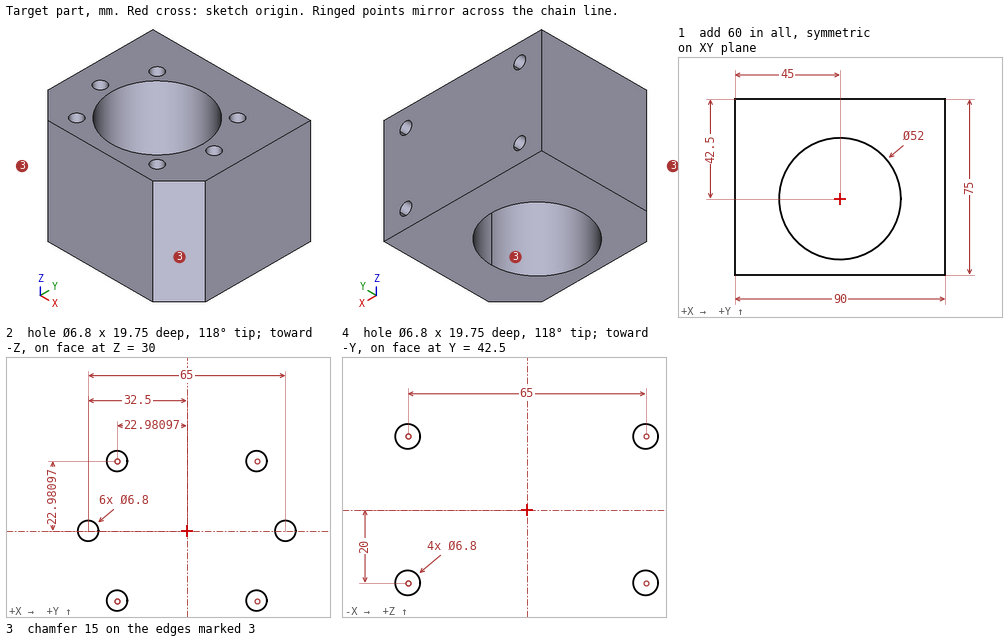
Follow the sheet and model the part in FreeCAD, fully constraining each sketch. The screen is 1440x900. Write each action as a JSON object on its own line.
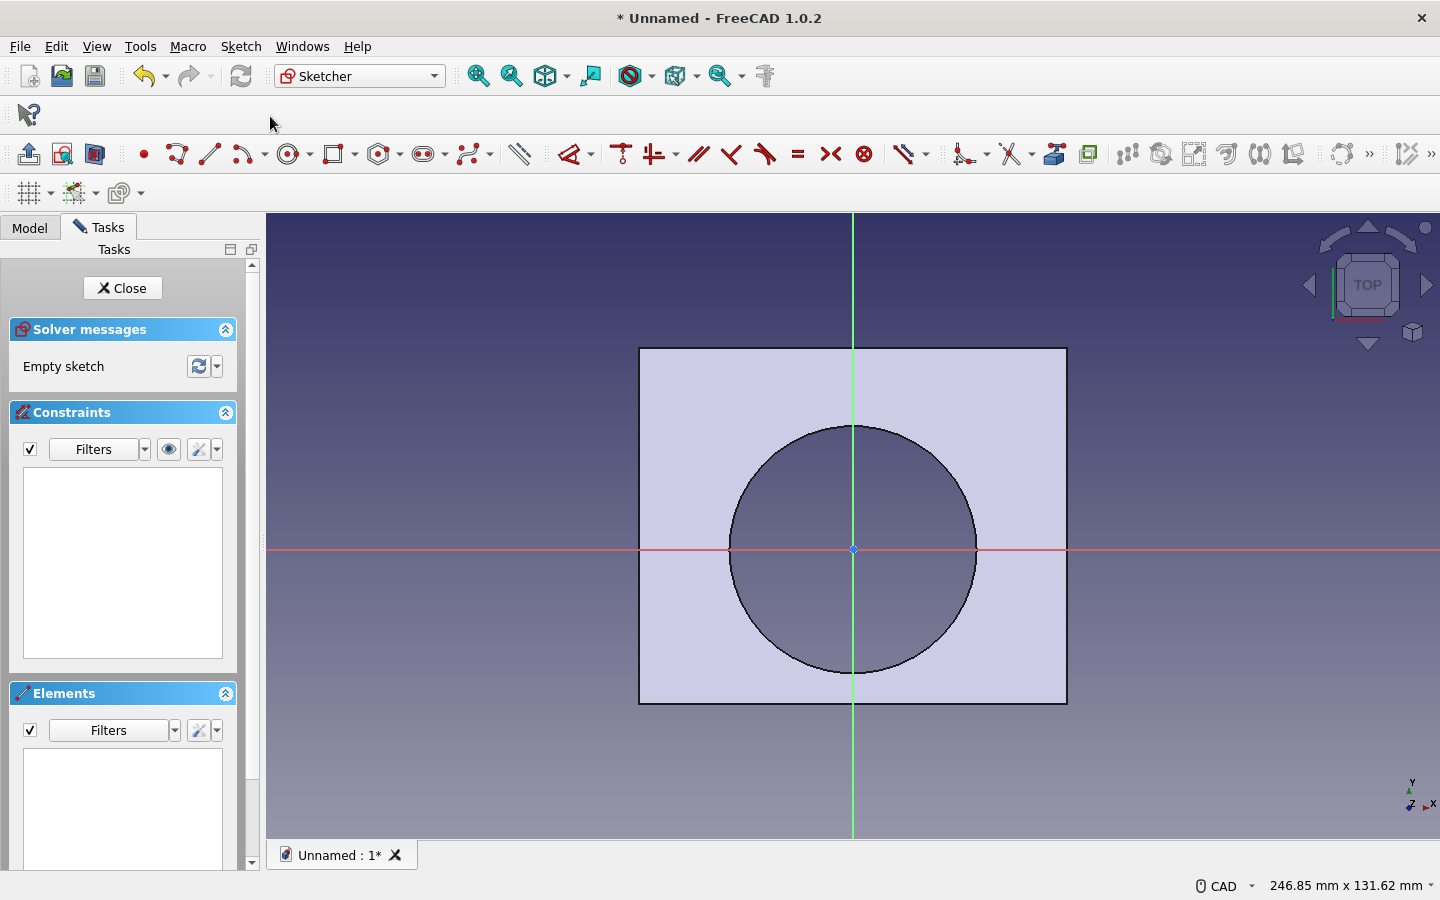
{"action": "scroll", "coordinate": [992, 598], "scroll_direction": "up", "scroll_amount": 2}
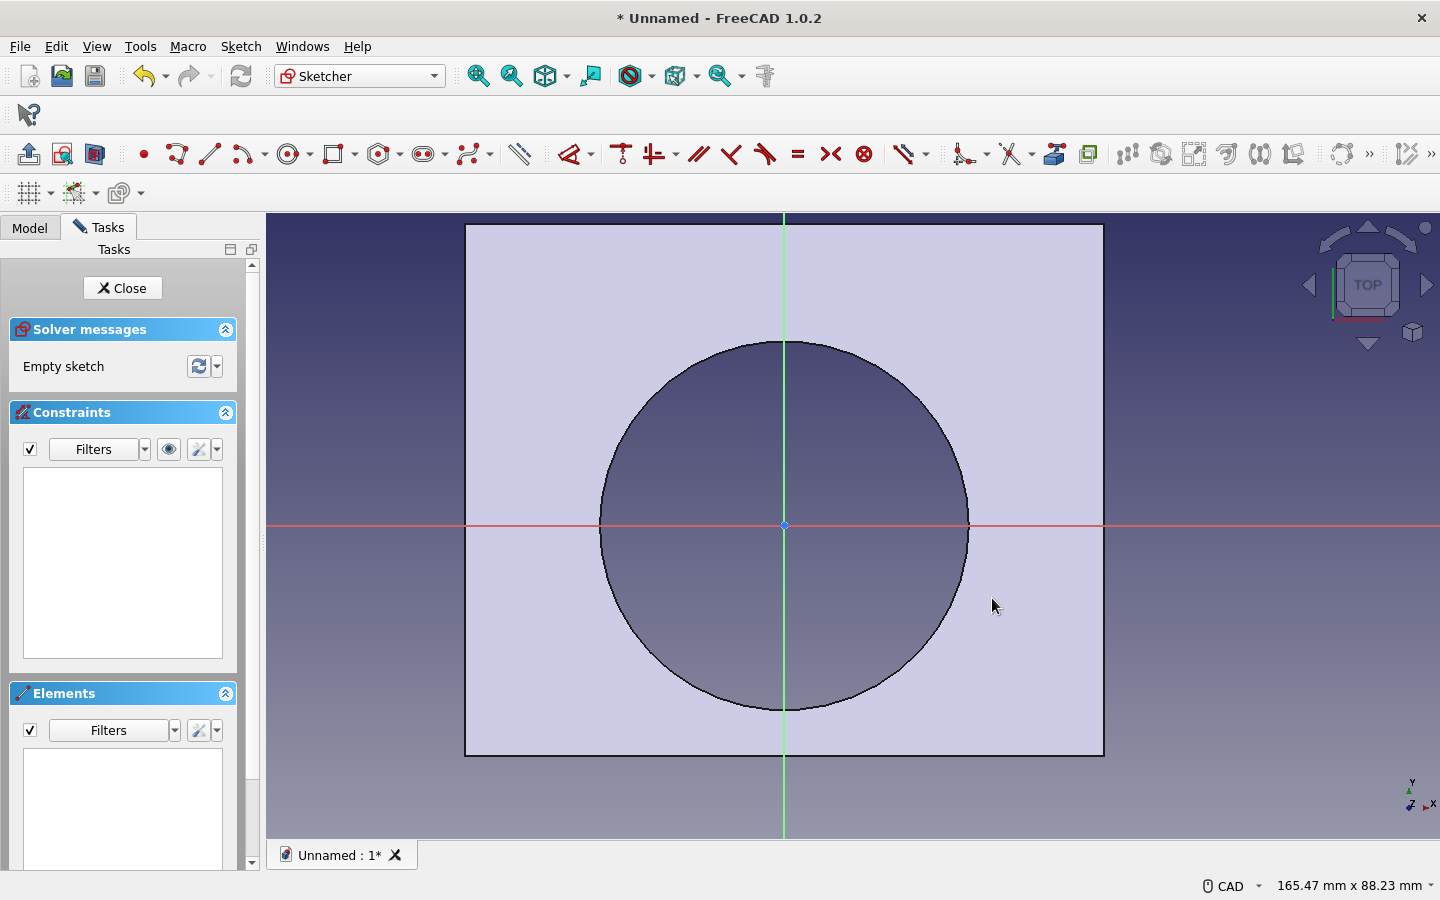
{"action": "left_click", "coordinate": [288, 154]}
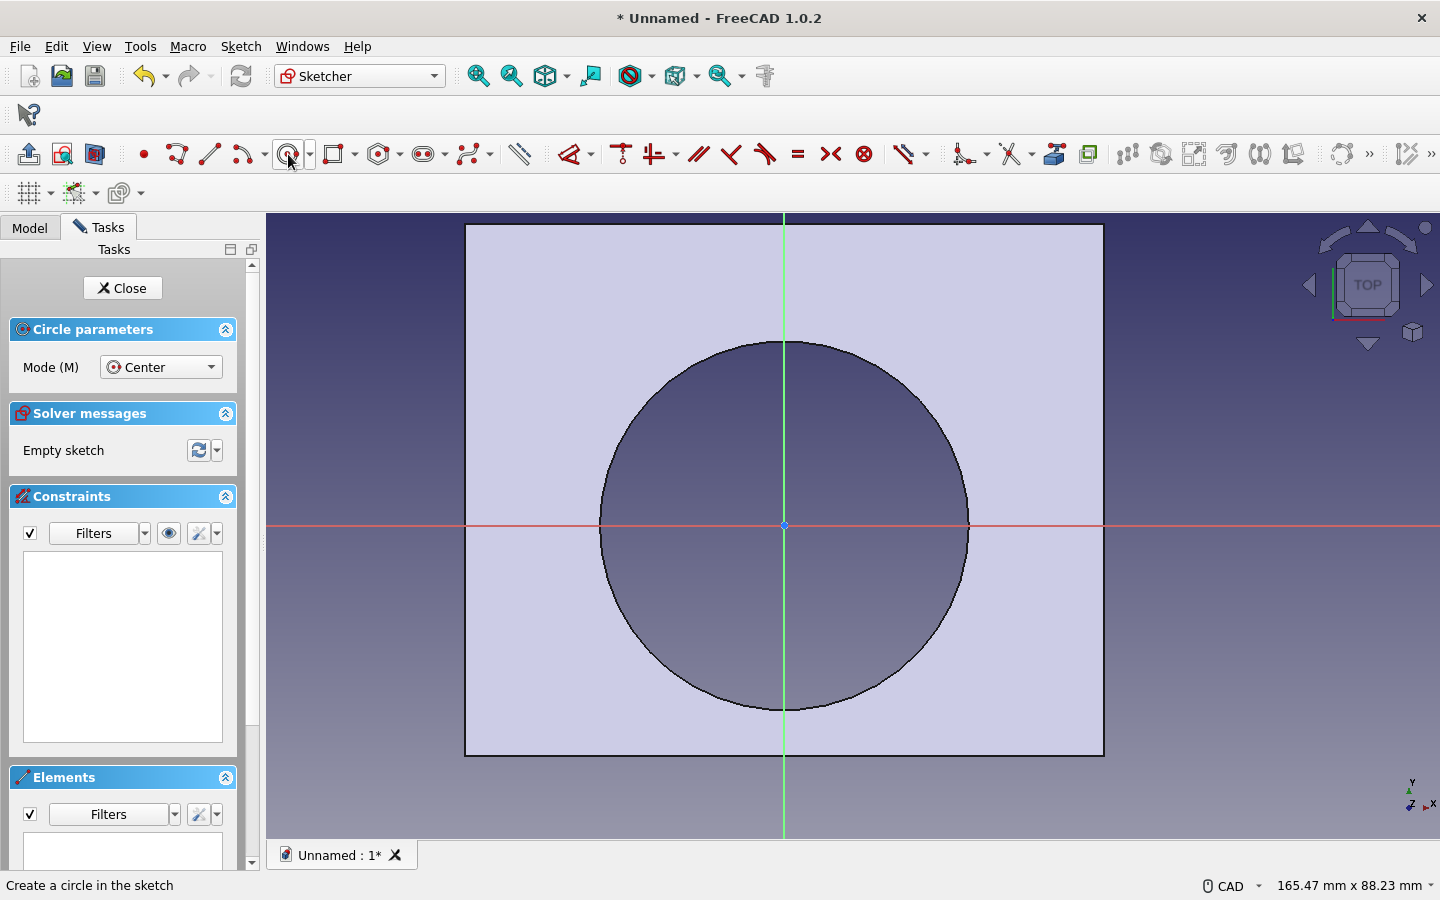
{"action": "left_click", "coordinate": [554, 526]}
{"action": "mouse_move", "coordinate": [571, 509]}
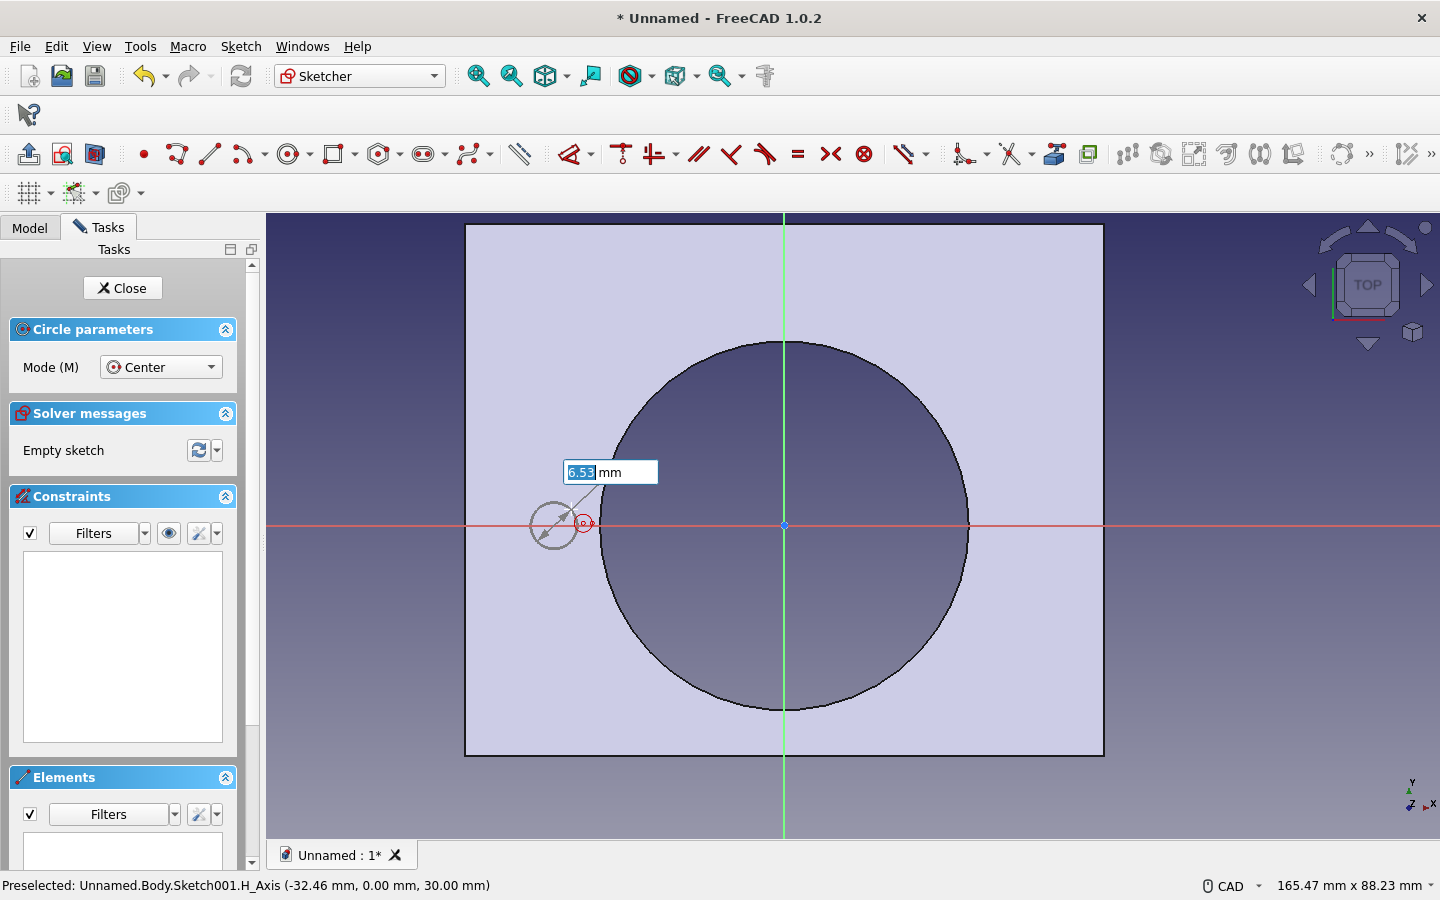
{"action": "type", "text": "6.8"}
{"action": "key", "text": "Return"}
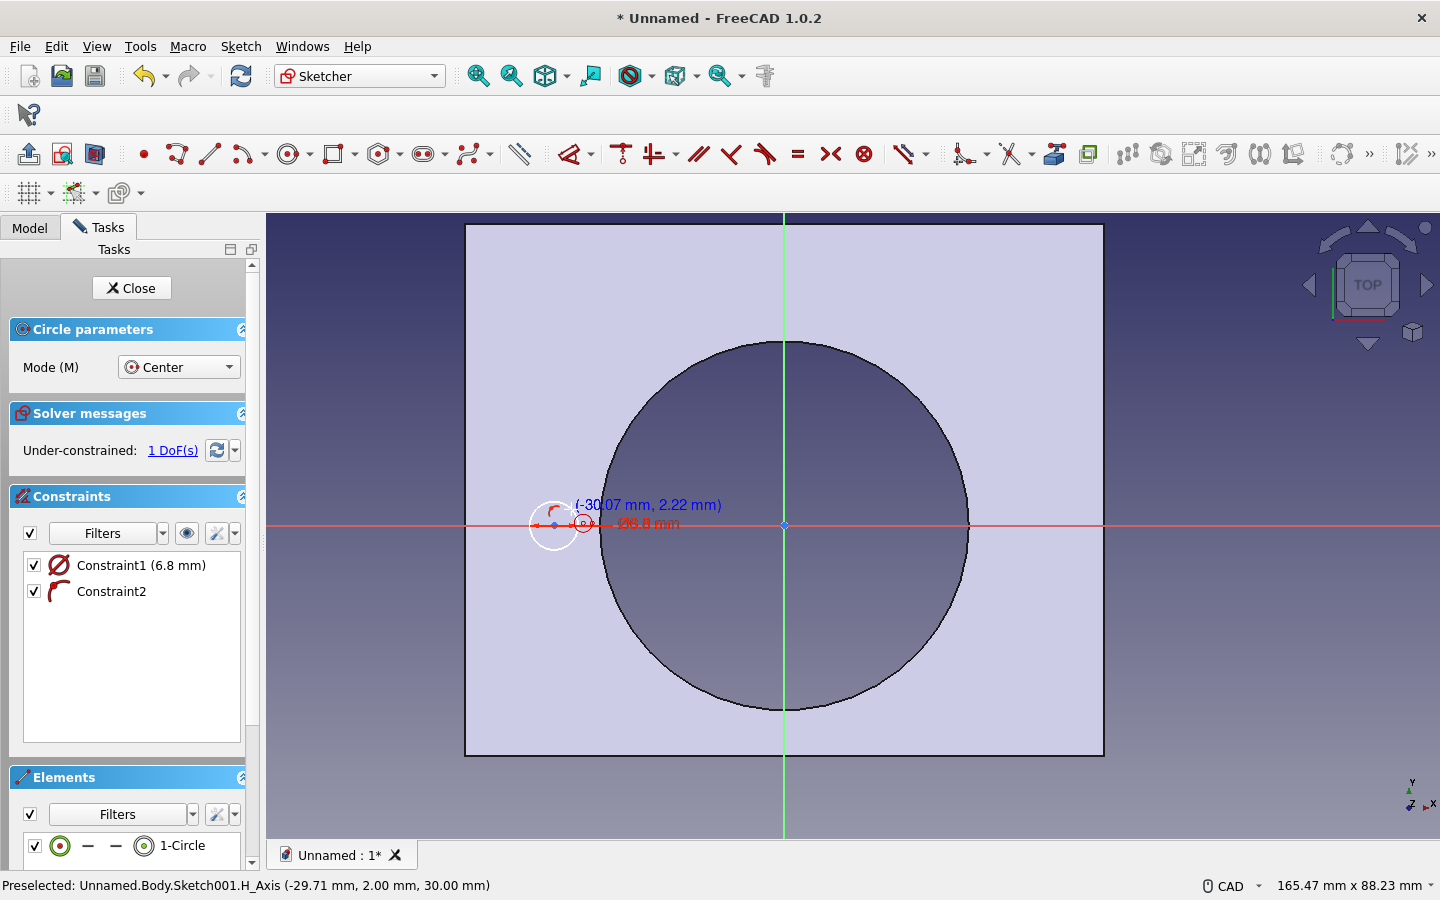
{"action": "left_click", "coordinate": [621, 363]}
{"action": "mouse_move", "coordinate": [638, 346]}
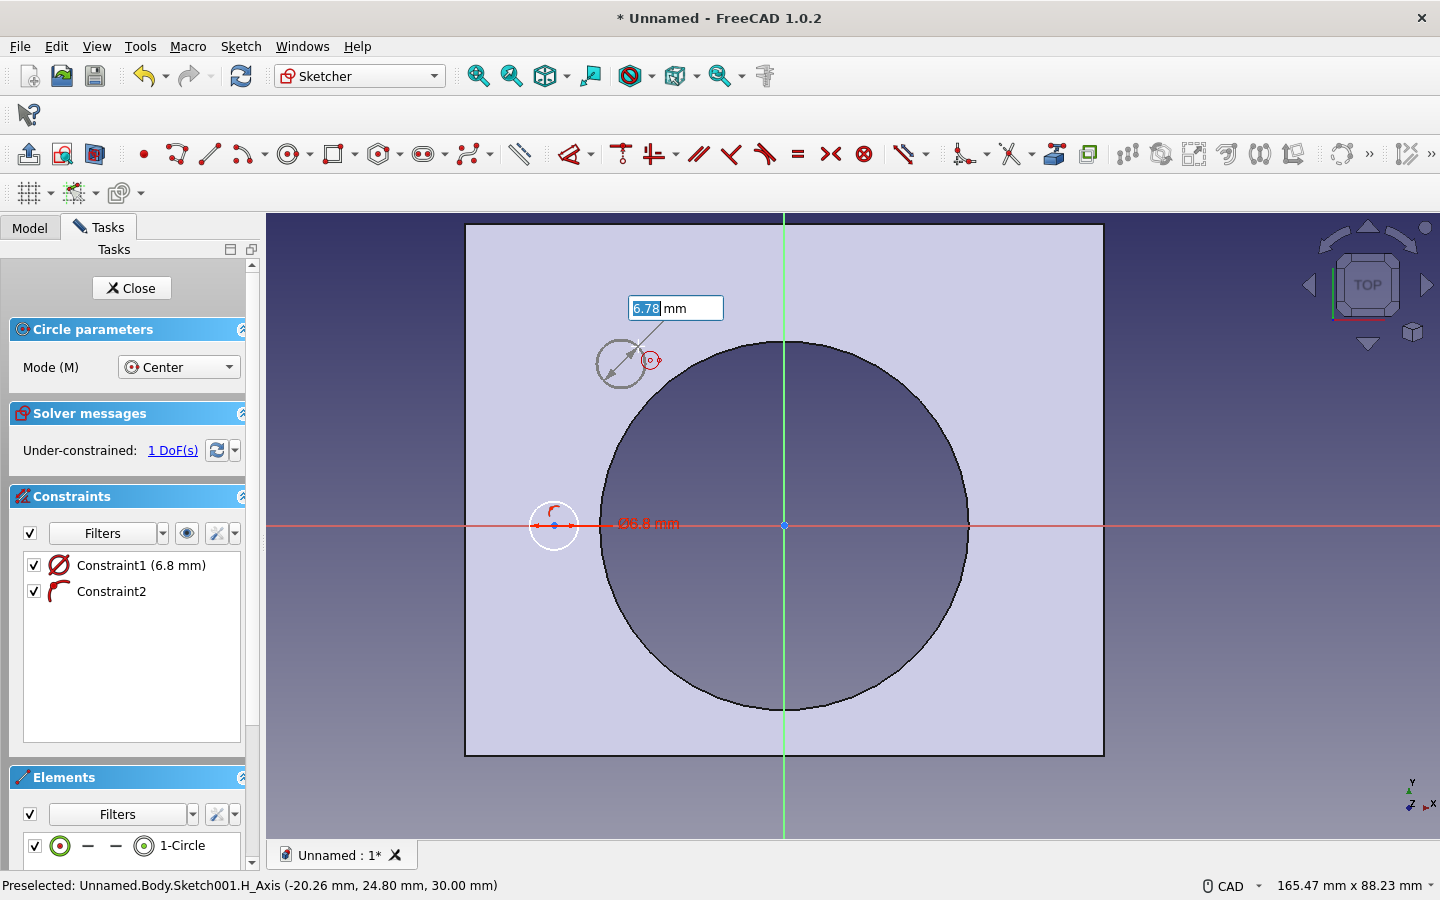
{"action": "type", "text": "6.8"}
{"action": "key", "text": "Return"}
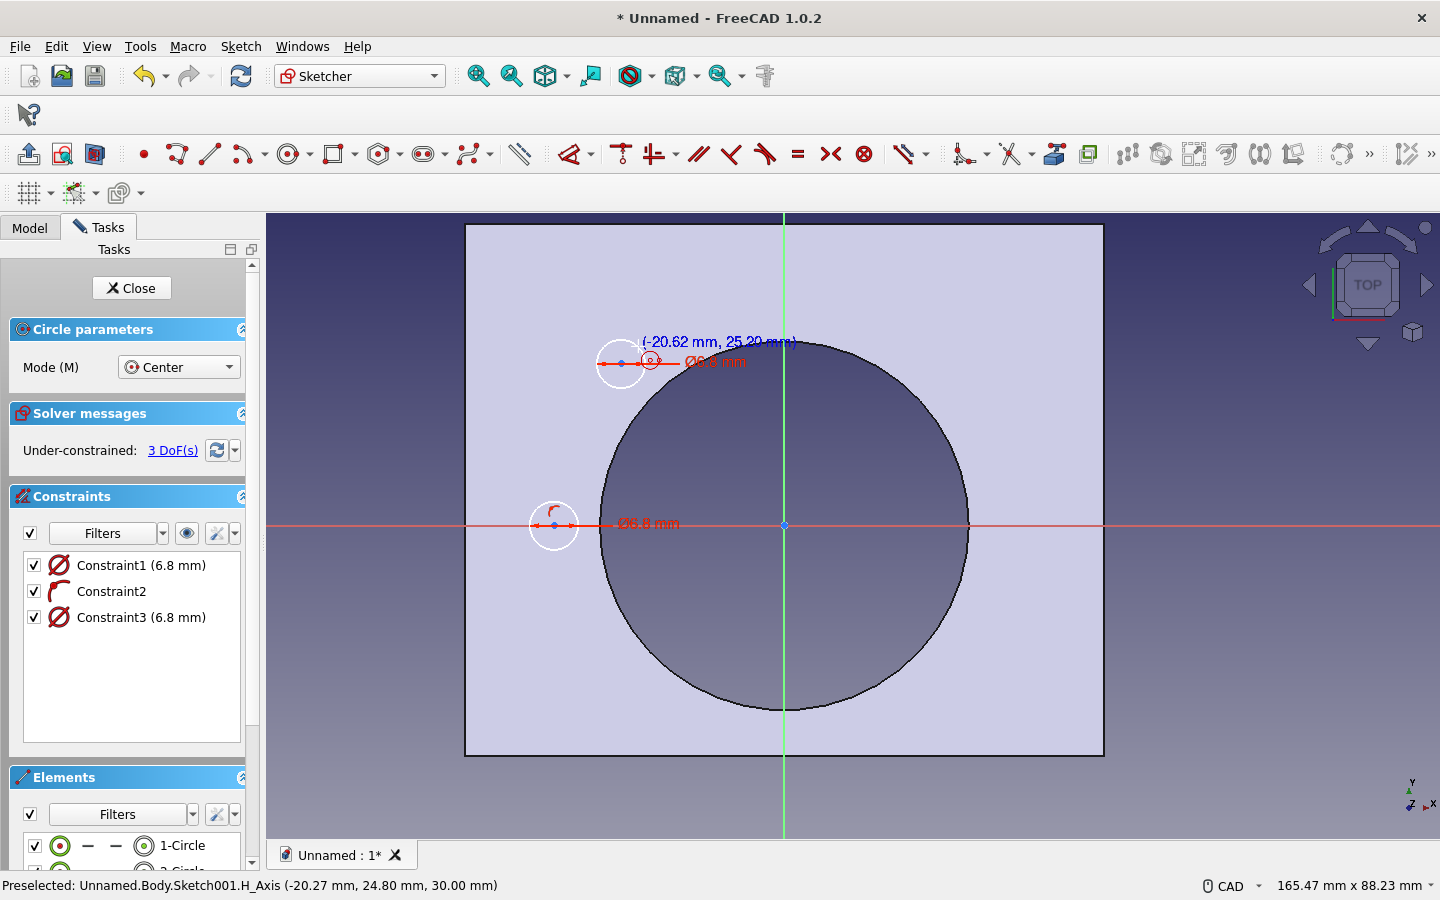
{"action": "left_click", "coordinate": [621, 689]}
{"action": "mouse_move", "coordinate": [638, 672]}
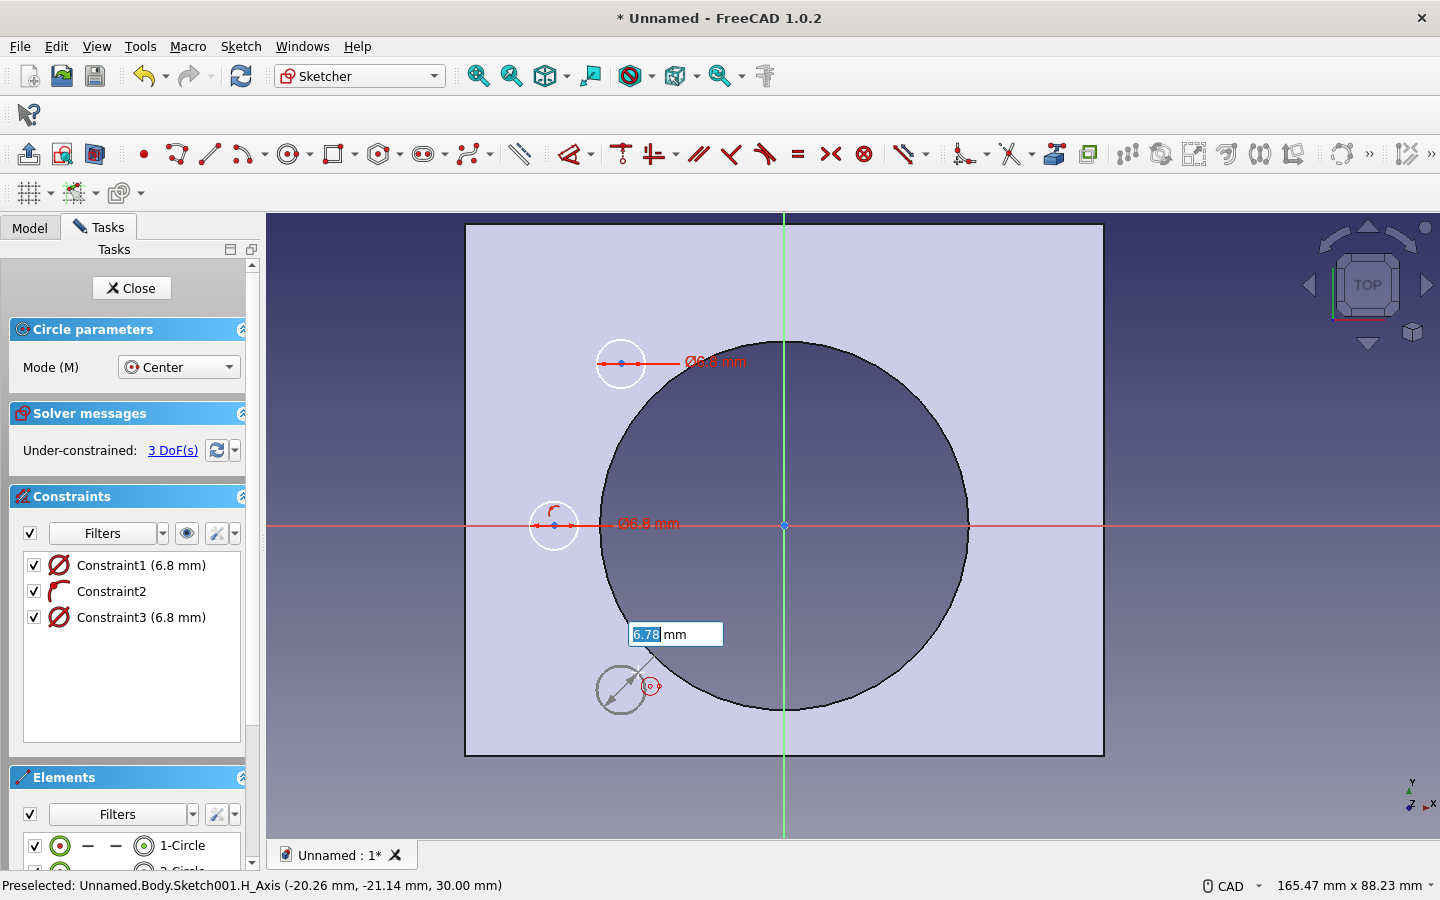
{"action": "type", "text": "6.8"}
{"action": "key", "text": "Return"}